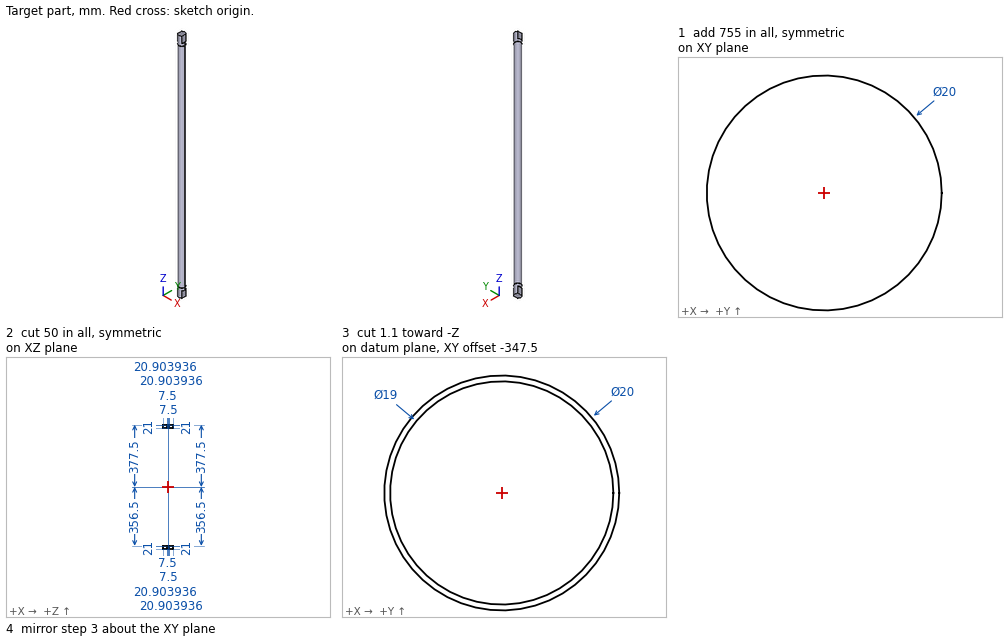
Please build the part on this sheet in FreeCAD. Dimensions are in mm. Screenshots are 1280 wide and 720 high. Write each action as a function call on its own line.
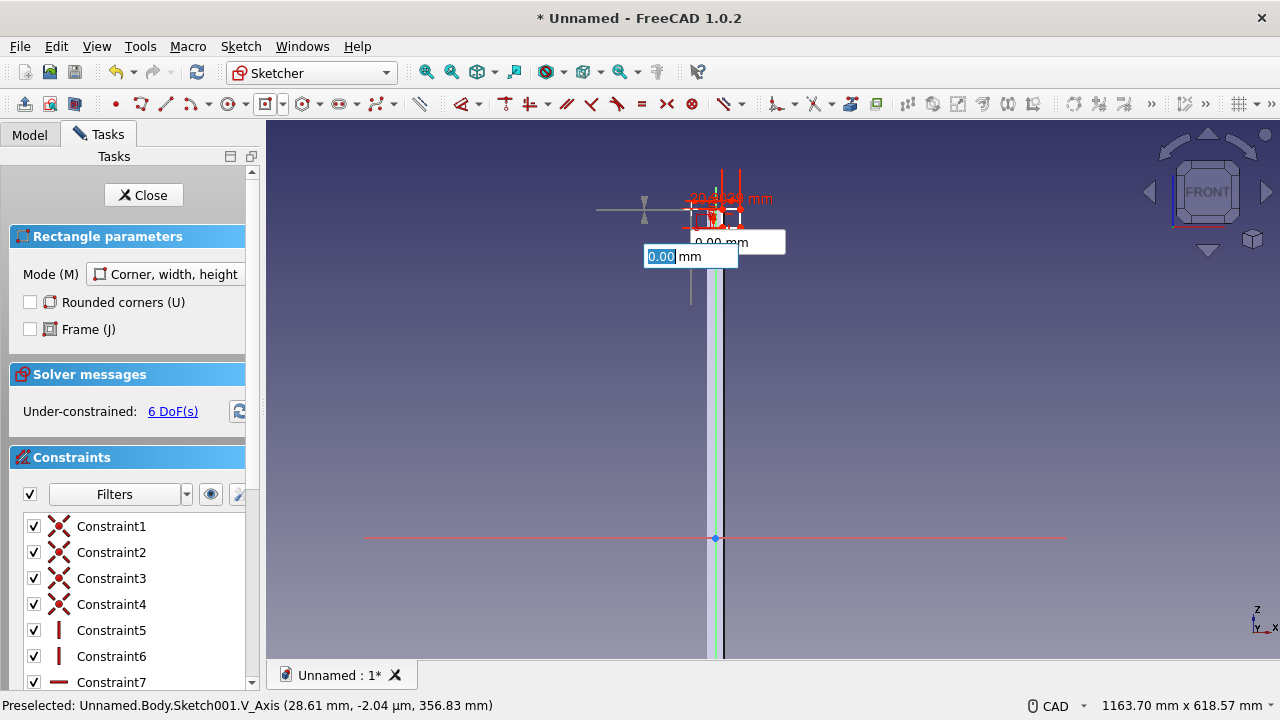
scroll(709, 227, up, 5)
move(708, 228)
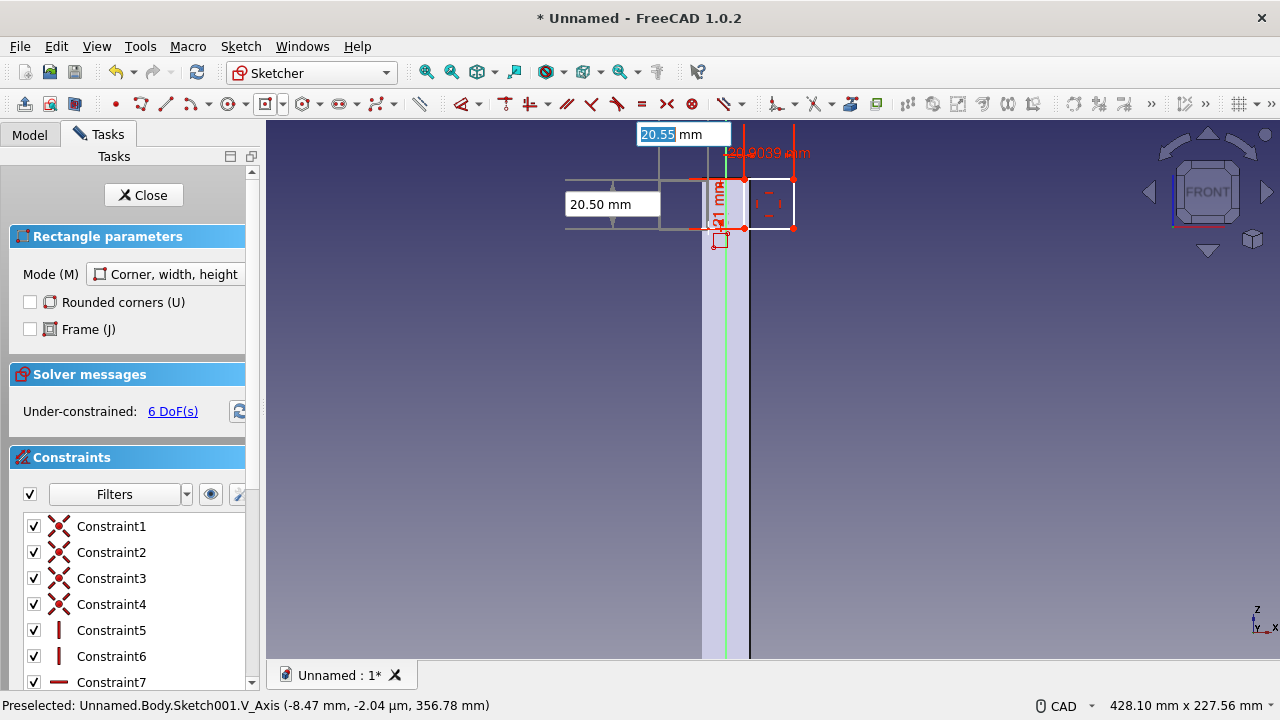
text(20.903936)
key(Tab)
text(21)
key(Return)
key(Escape)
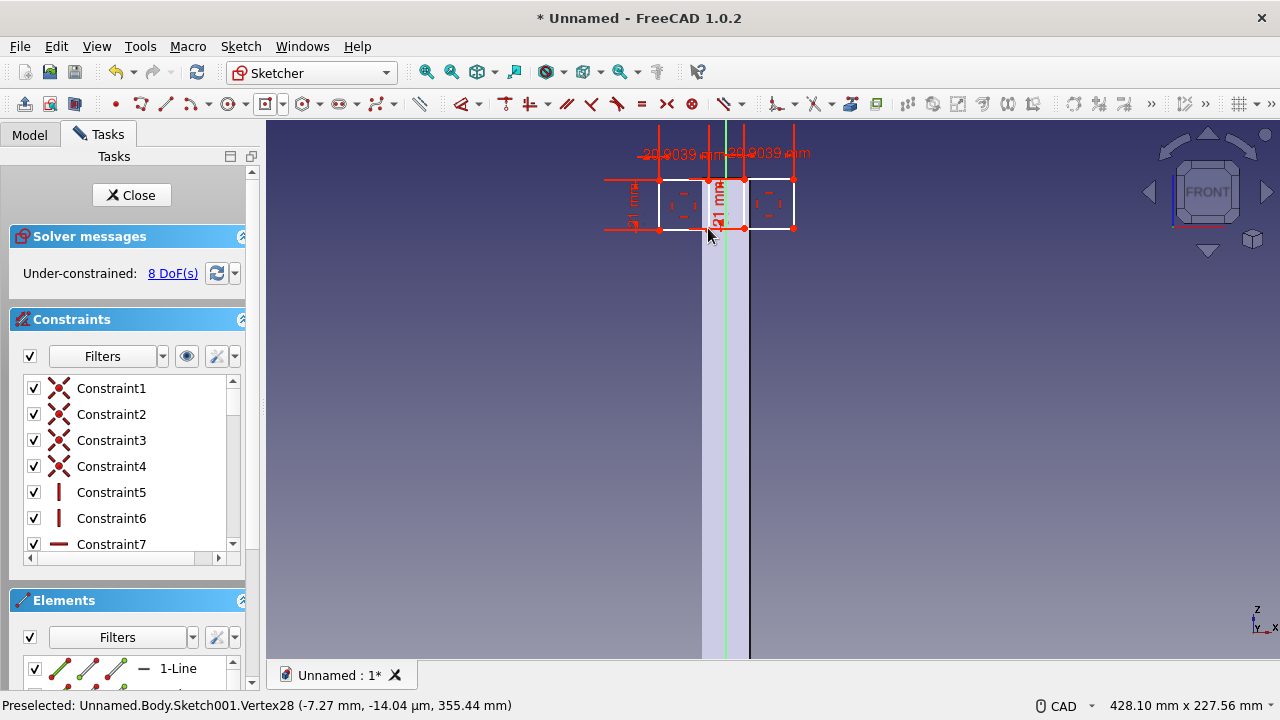
scroll(699, 217, down, 8)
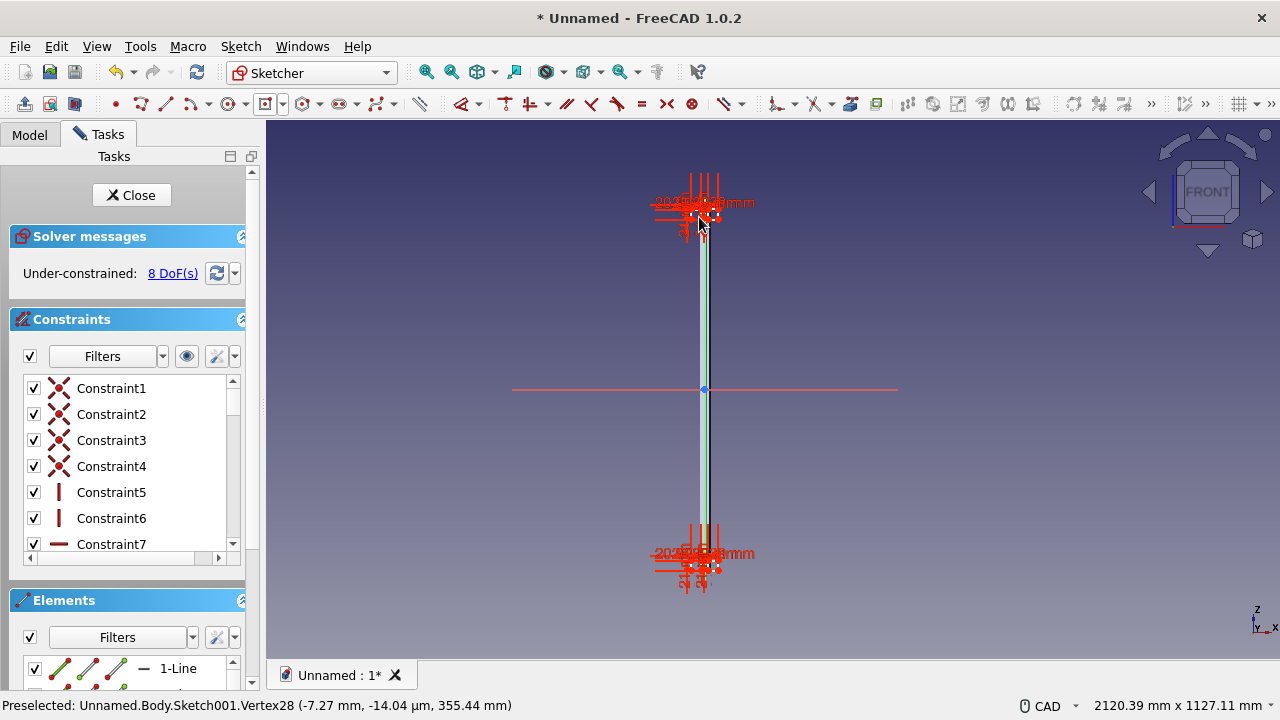
scroll(701, 571, up, 13)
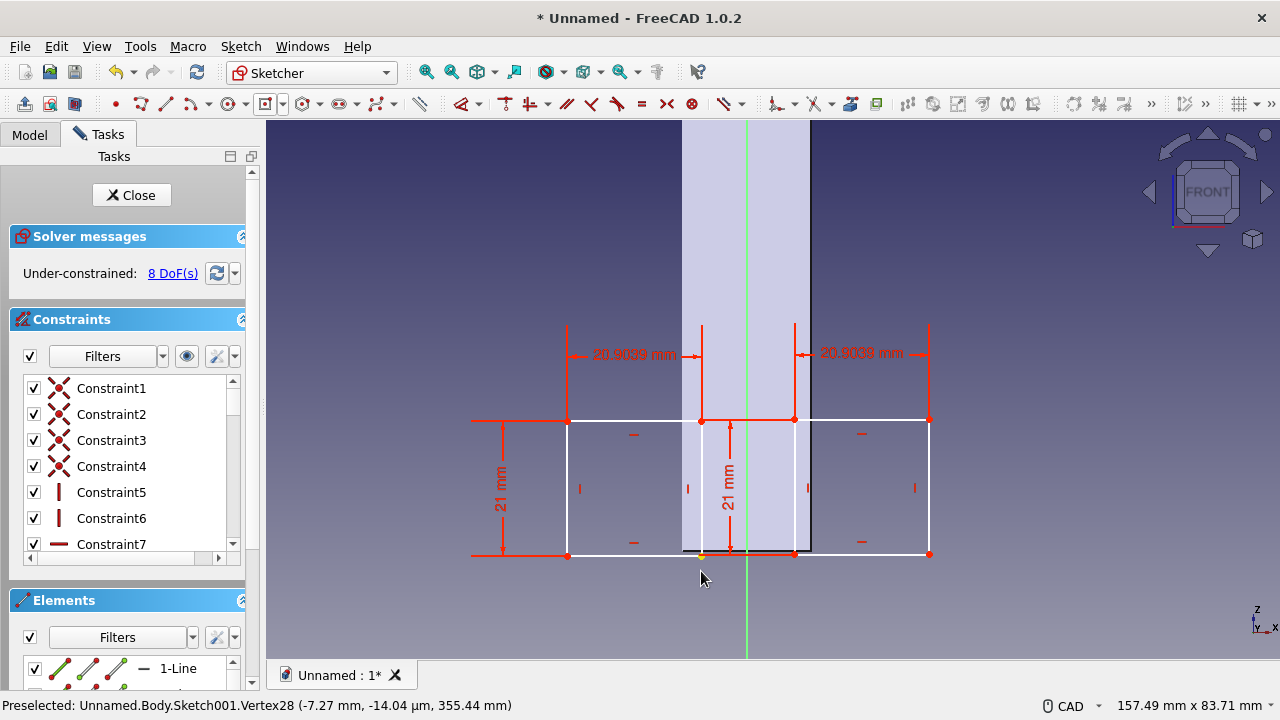
click(702, 556)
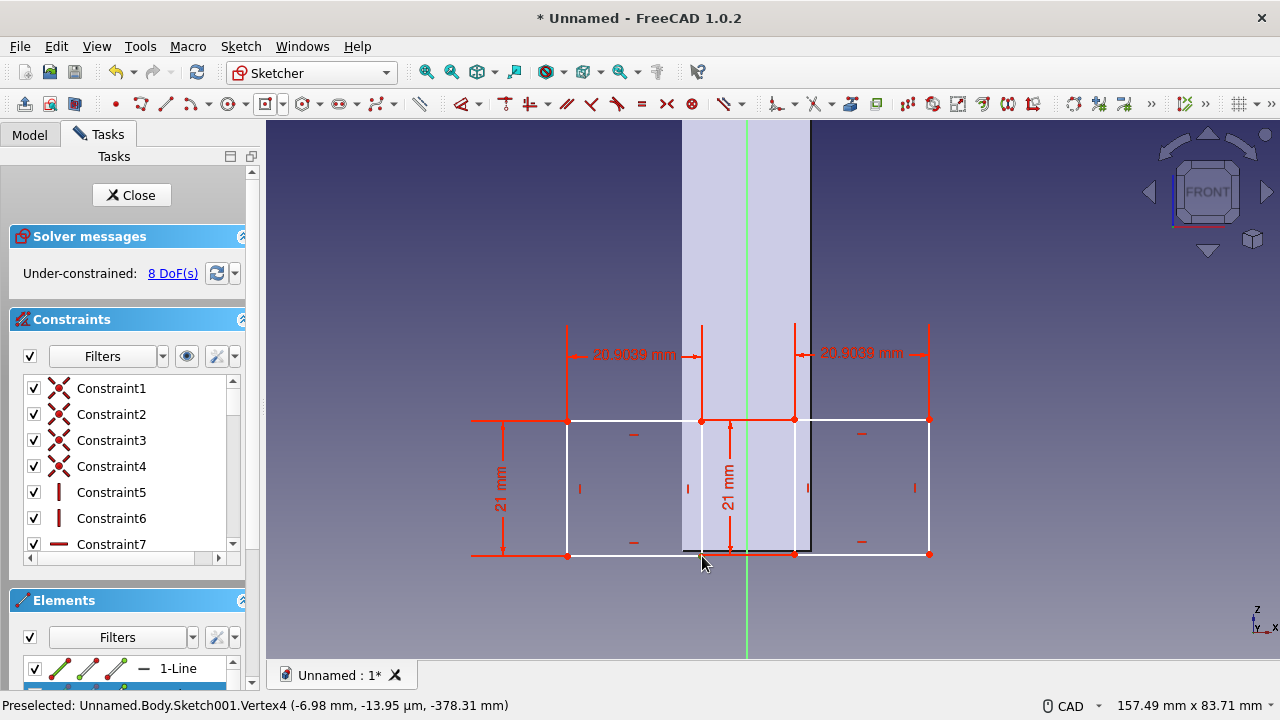
key(l)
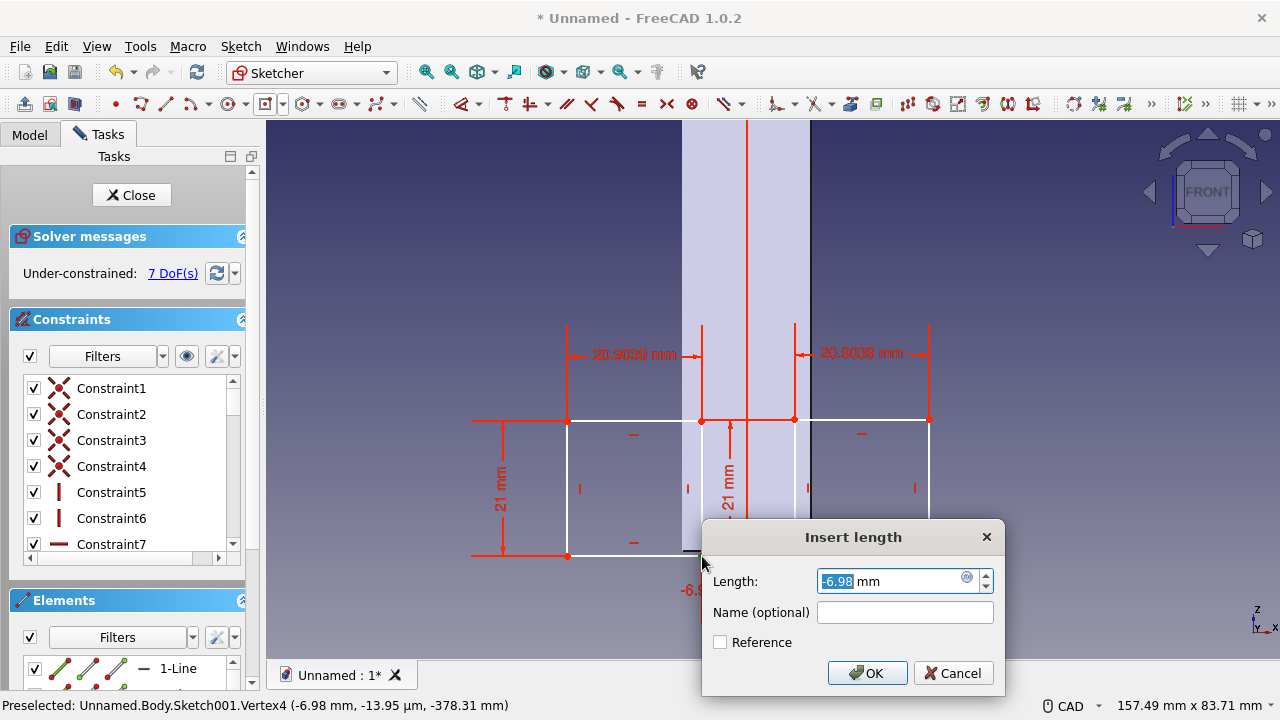
text(-7.5)
key(Return)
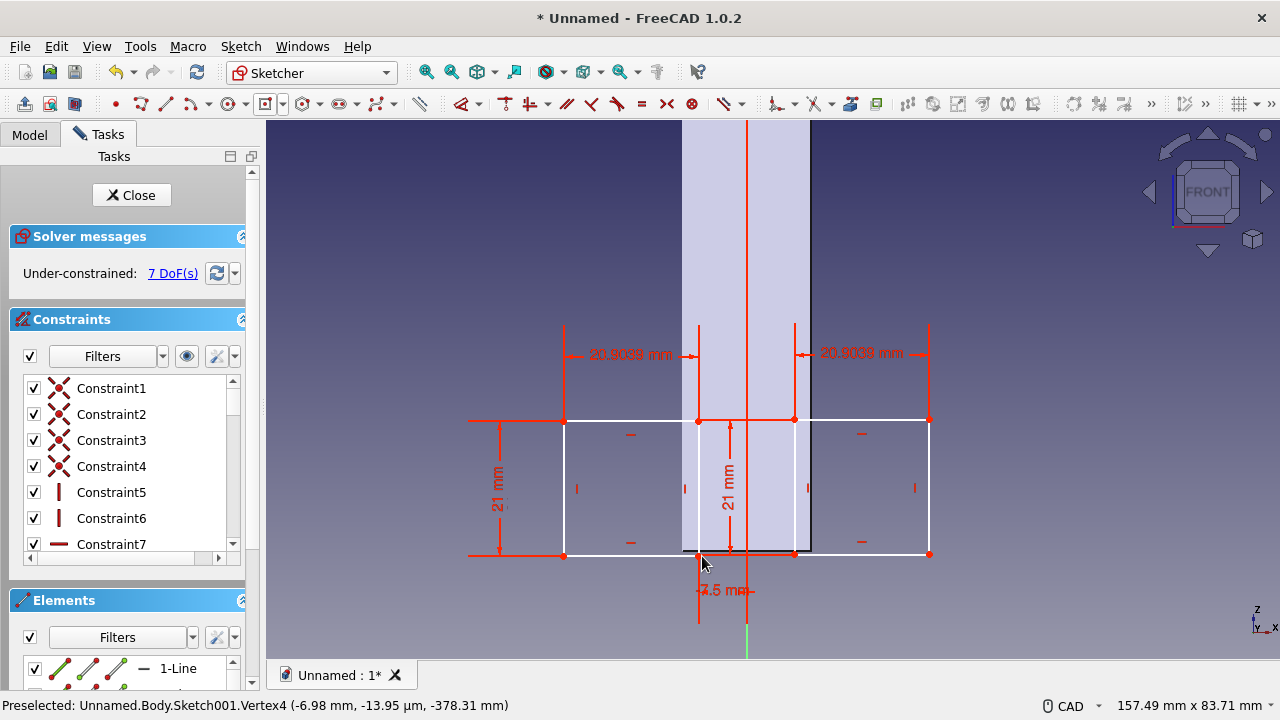
click(795, 420)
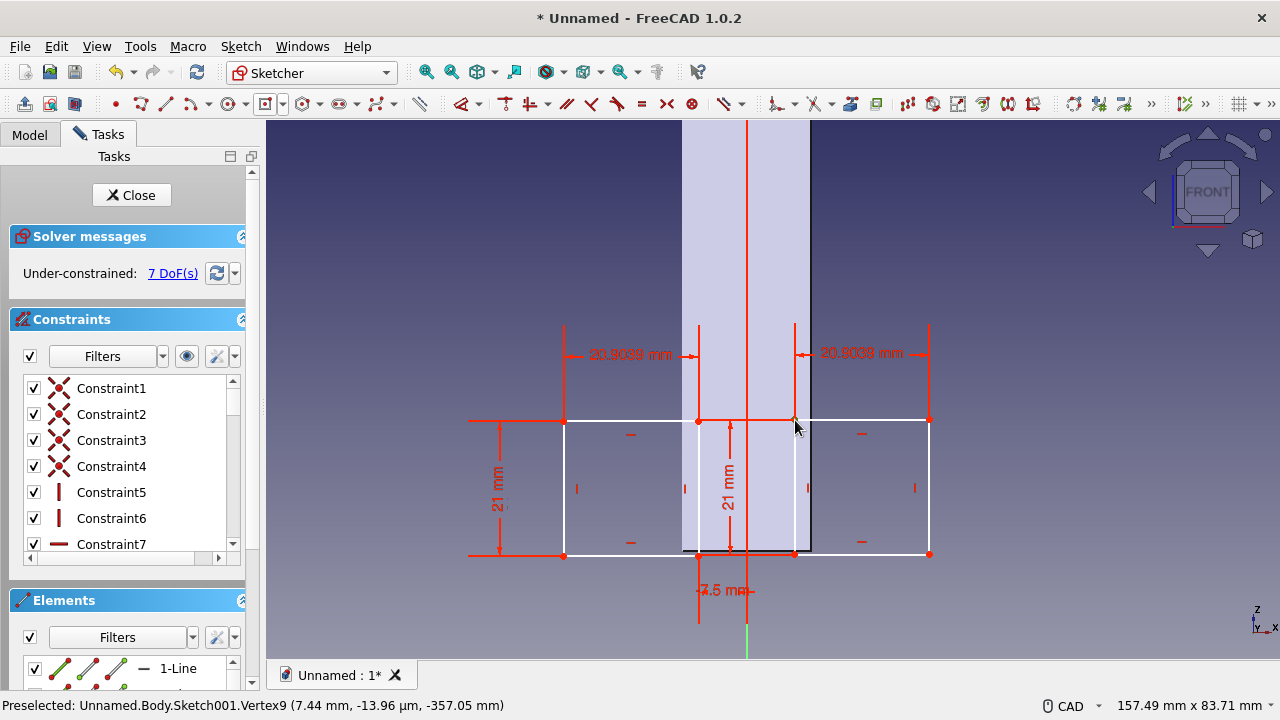
key(l)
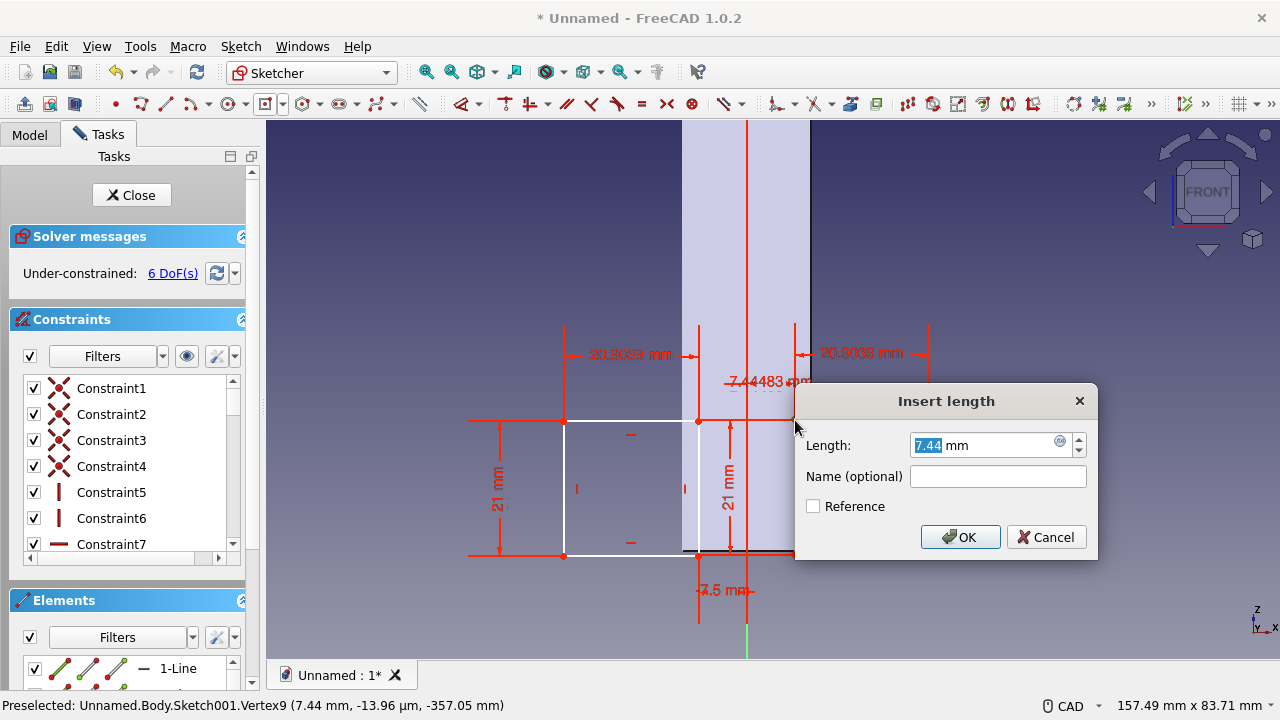
text(7.5)
key(Return)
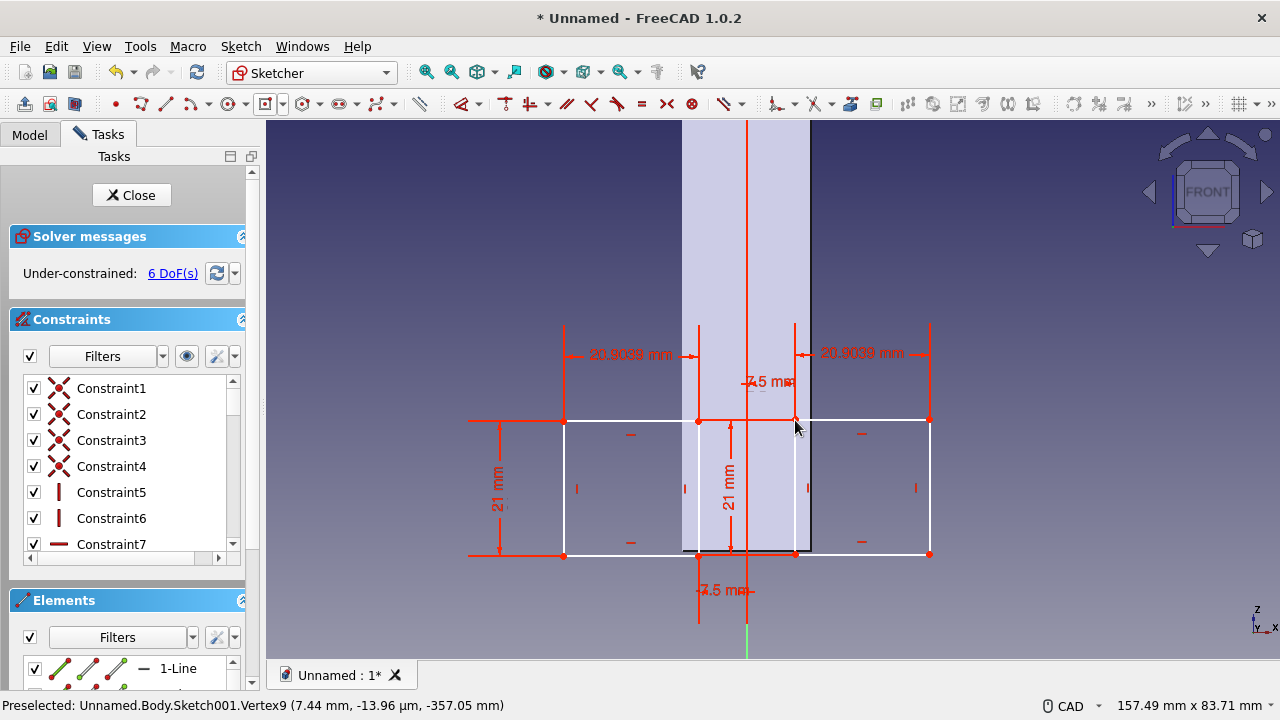
scroll(701, 572, down, 13)